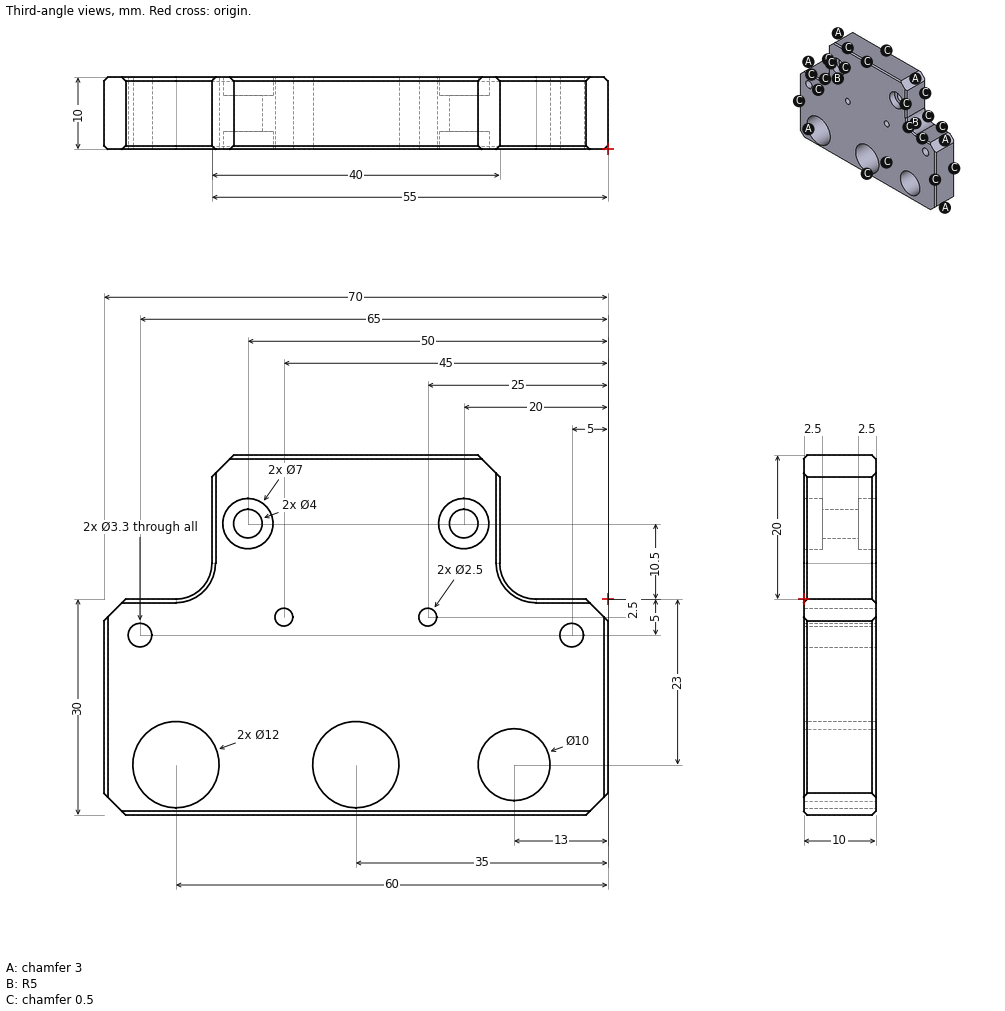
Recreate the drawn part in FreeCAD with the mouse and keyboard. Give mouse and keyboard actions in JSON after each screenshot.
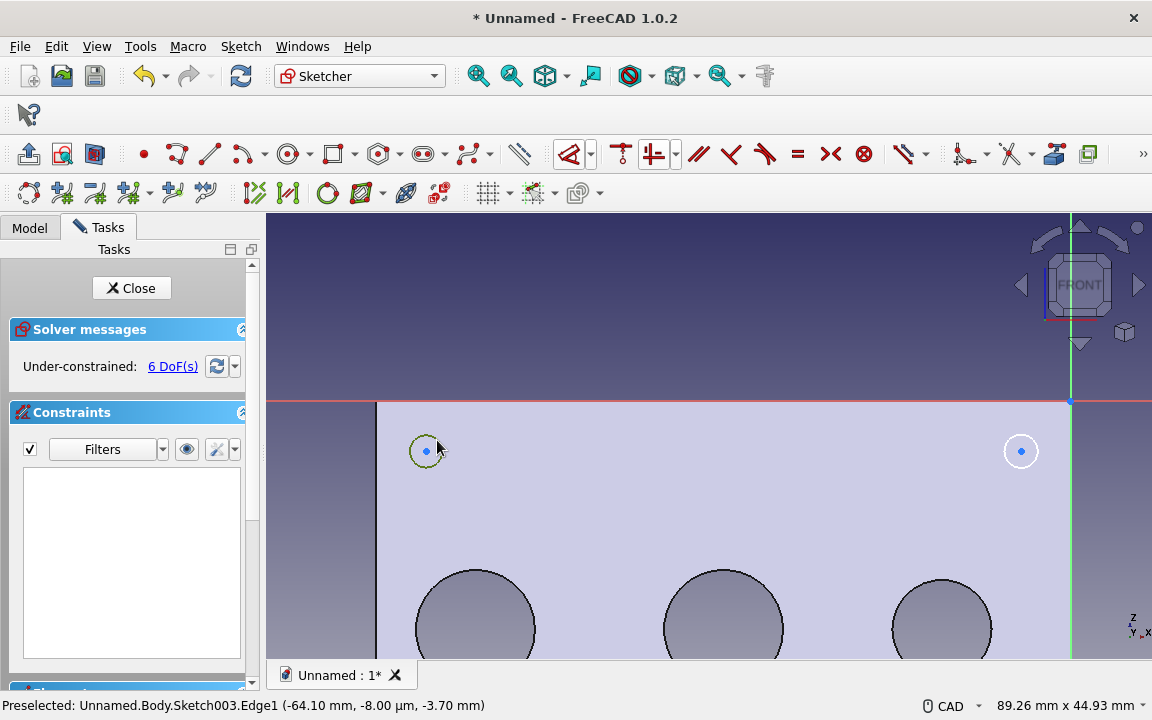
{"action": "scroll", "coordinate": [438, 440], "scroll_direction": "down", "scroll_amount": 2}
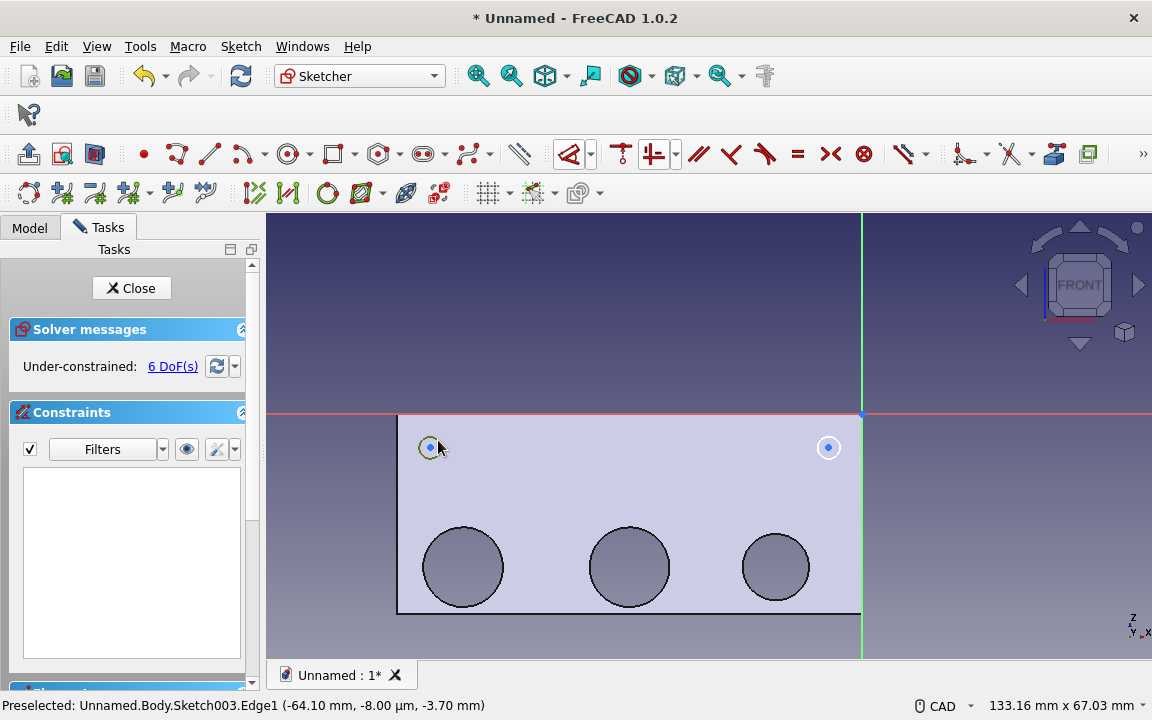
{"action": "scroll", "coordinate": [837, 440], "scroll_direction": "up", "scroll_amount": 2}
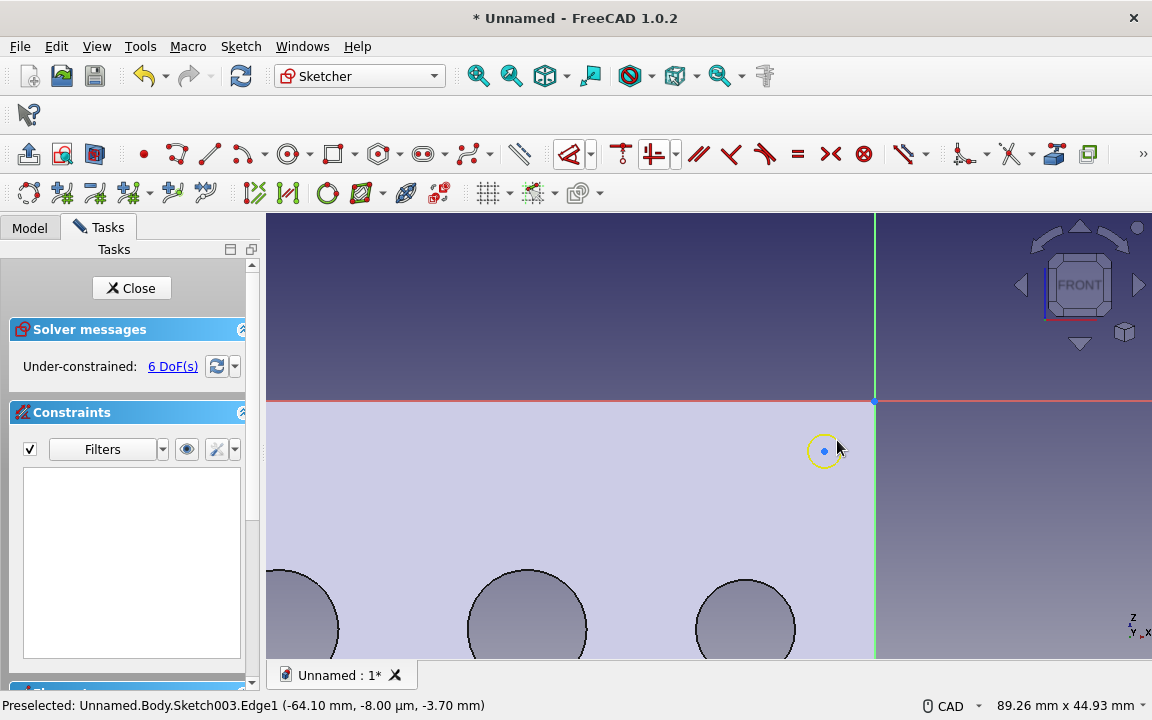
{"action": "left_click", "coordinate": [836, 440]}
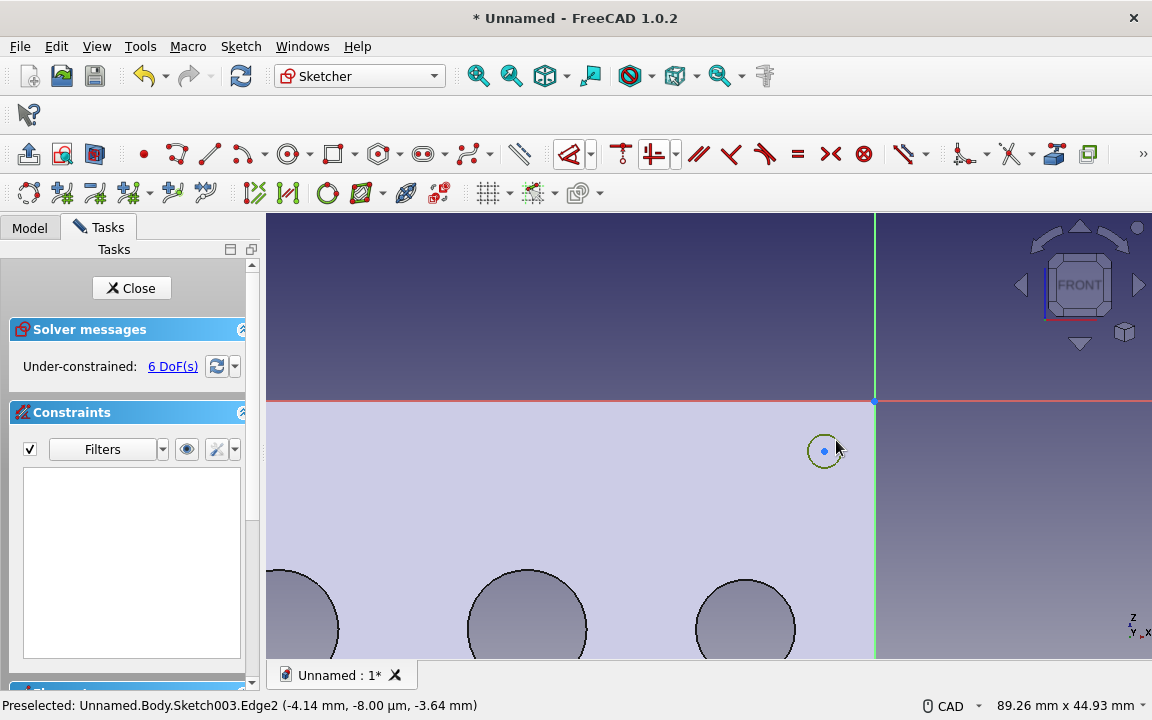
{"action": "left_click", "coordinate": [798, 154]}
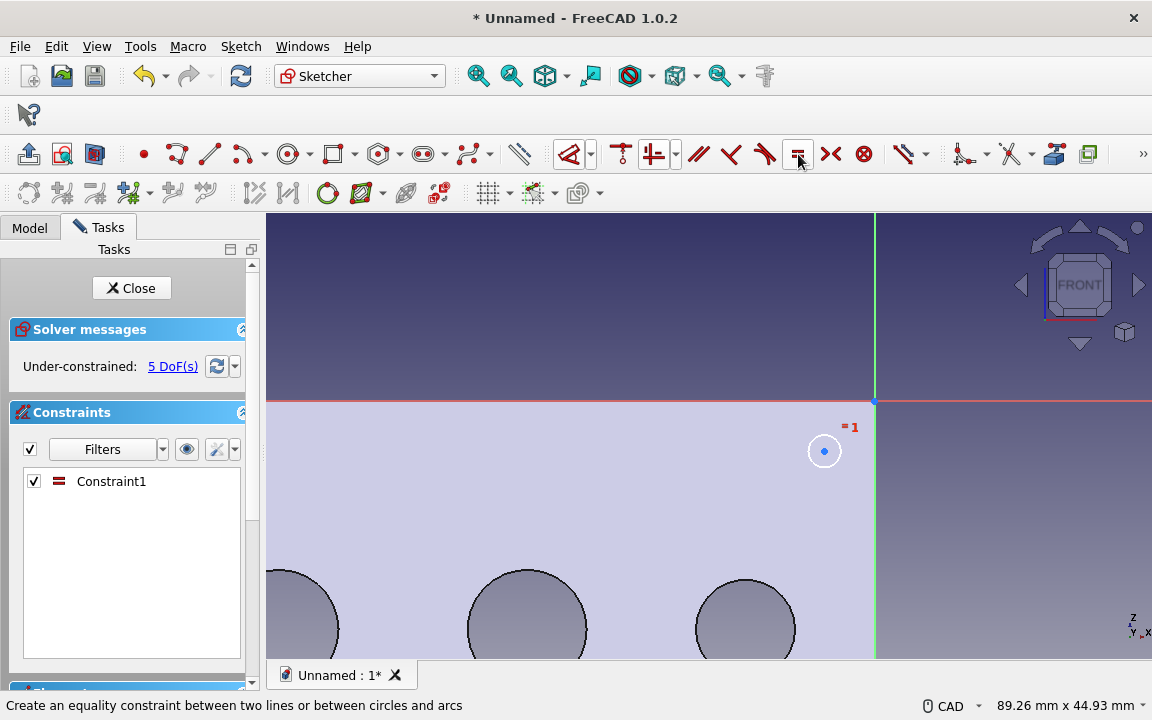
{"action": "scroll", "coordinate": [837, 440], "scroll_direction": "down", "scroll_amount": 2}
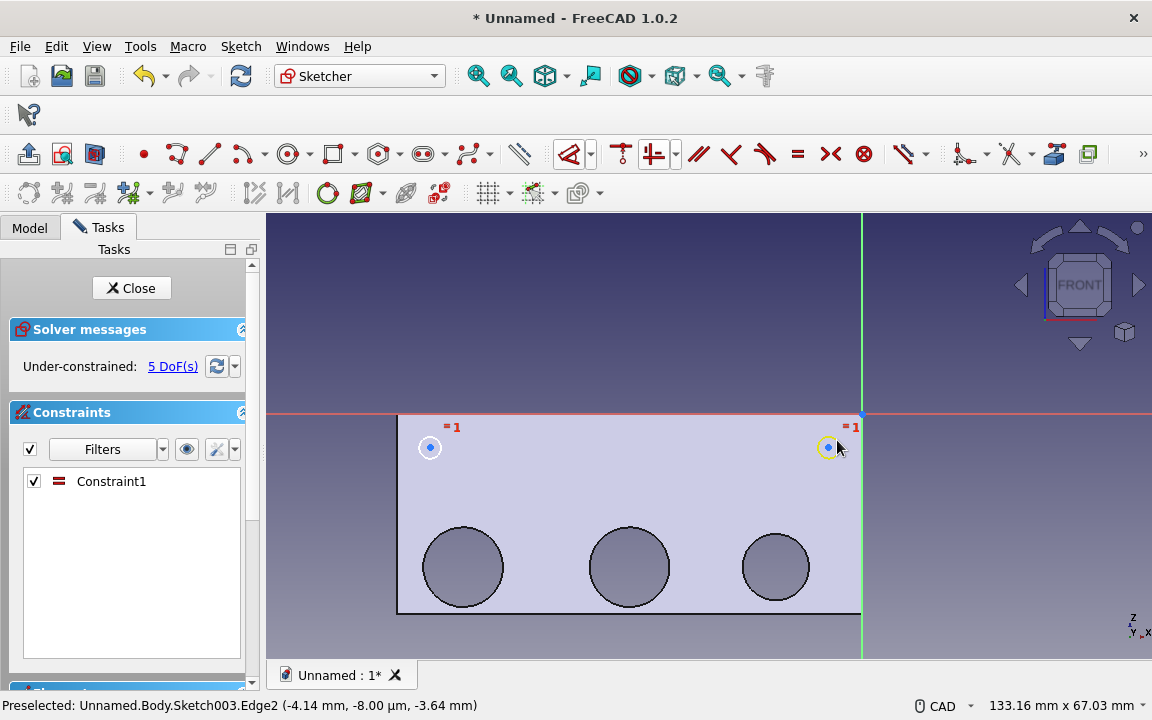
{"action": "left_click", "coordinate": [430, 448]}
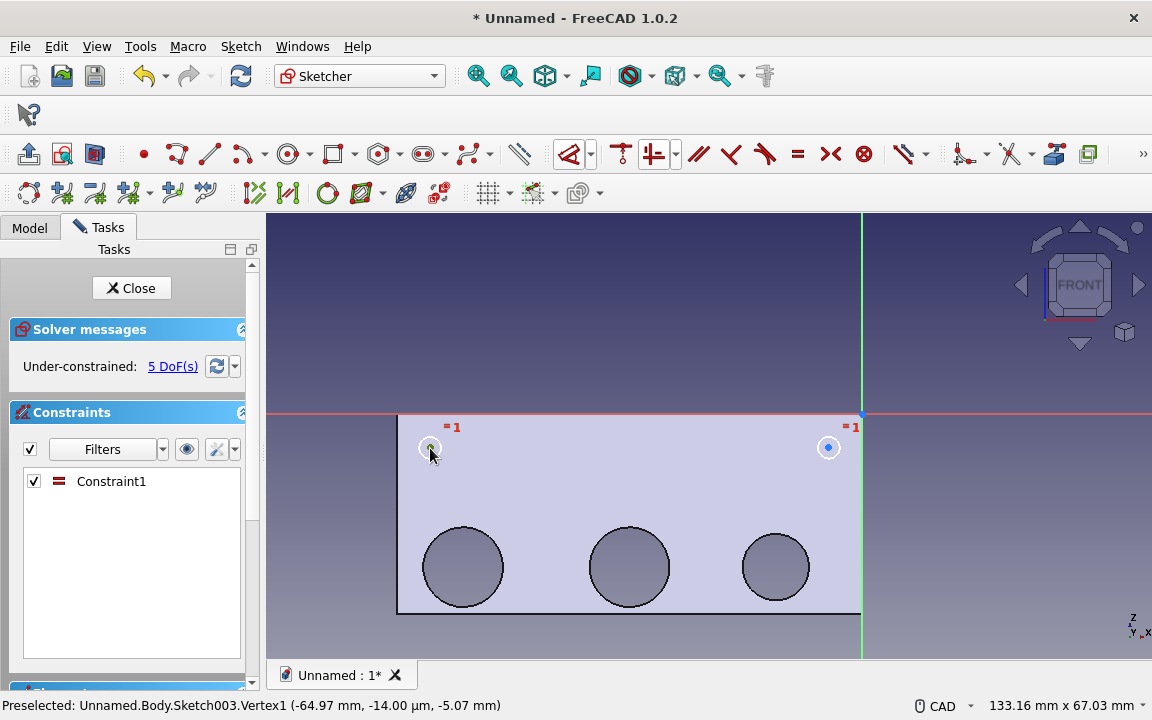
{"action": "left_click", "coordinate": [829, 448]}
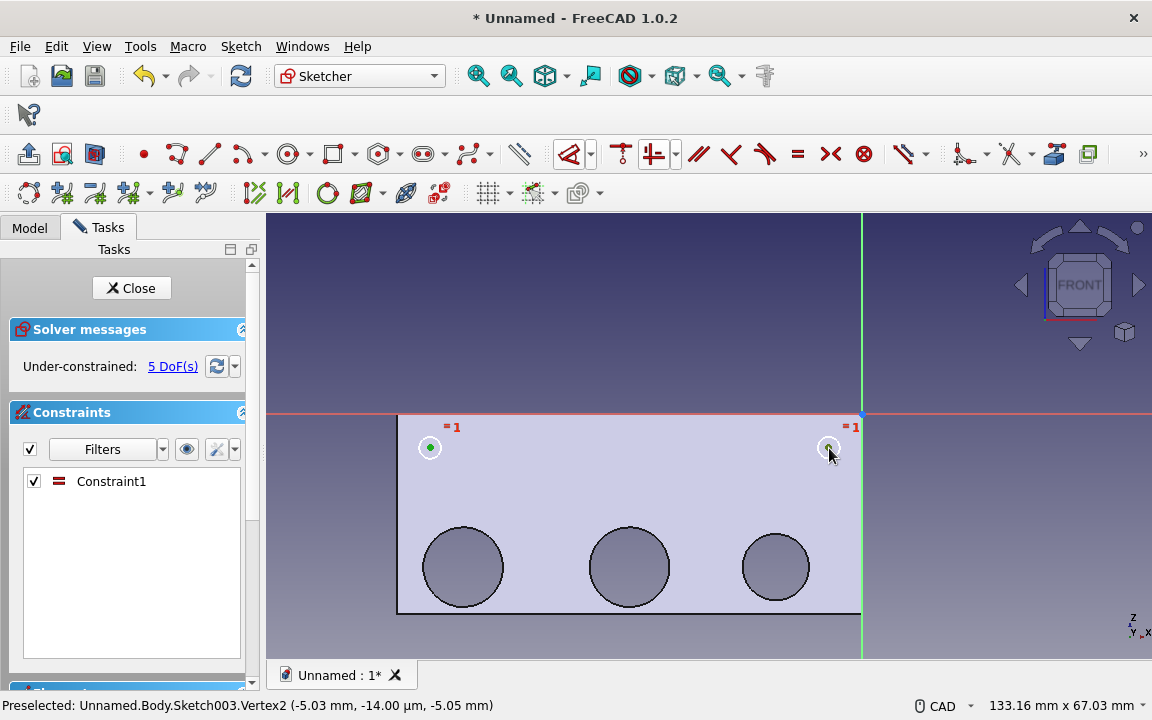
{"action": "left_click", "coordinate": [676, 154]}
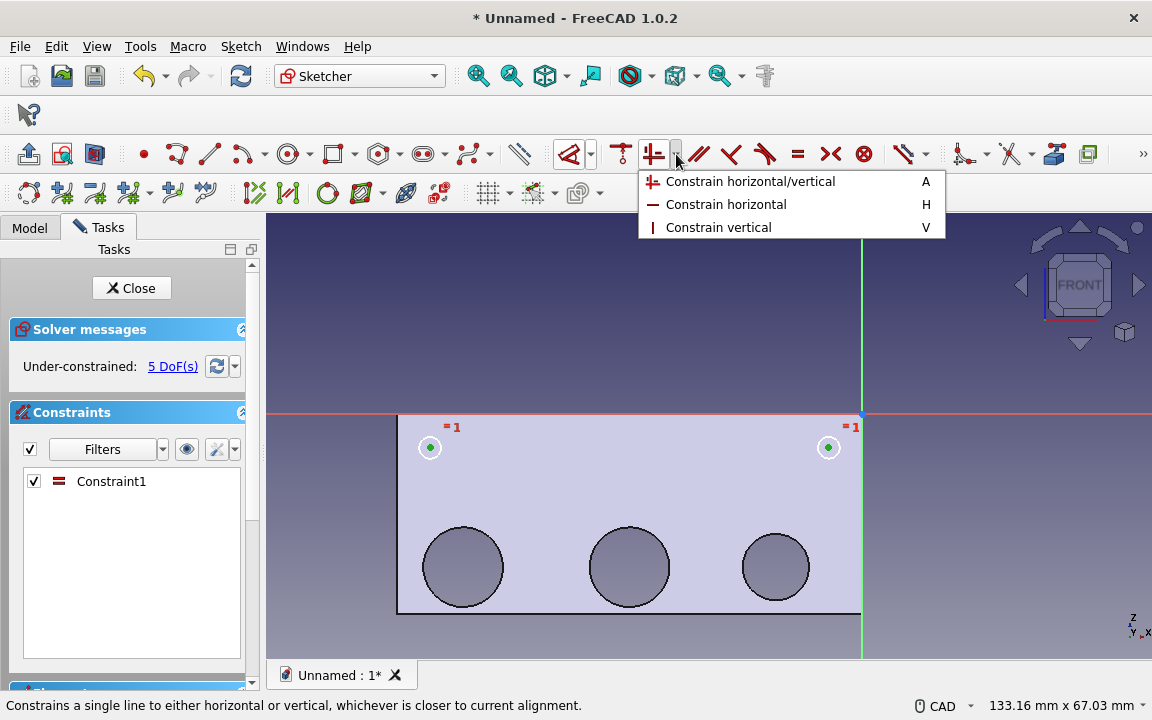
{"action": "left_click", "coordinate": [792, 204]}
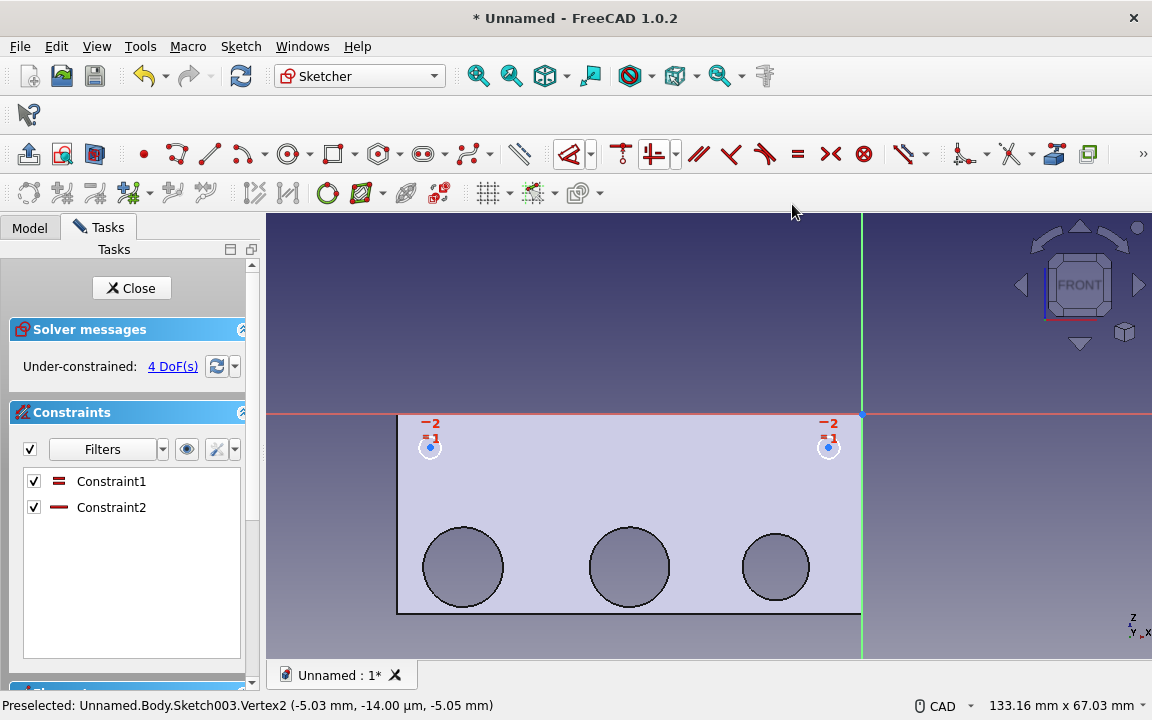
{"action": "scroll", "coordinate": [438, 440], "scroll_direction": "up", "scroll_amount": 3}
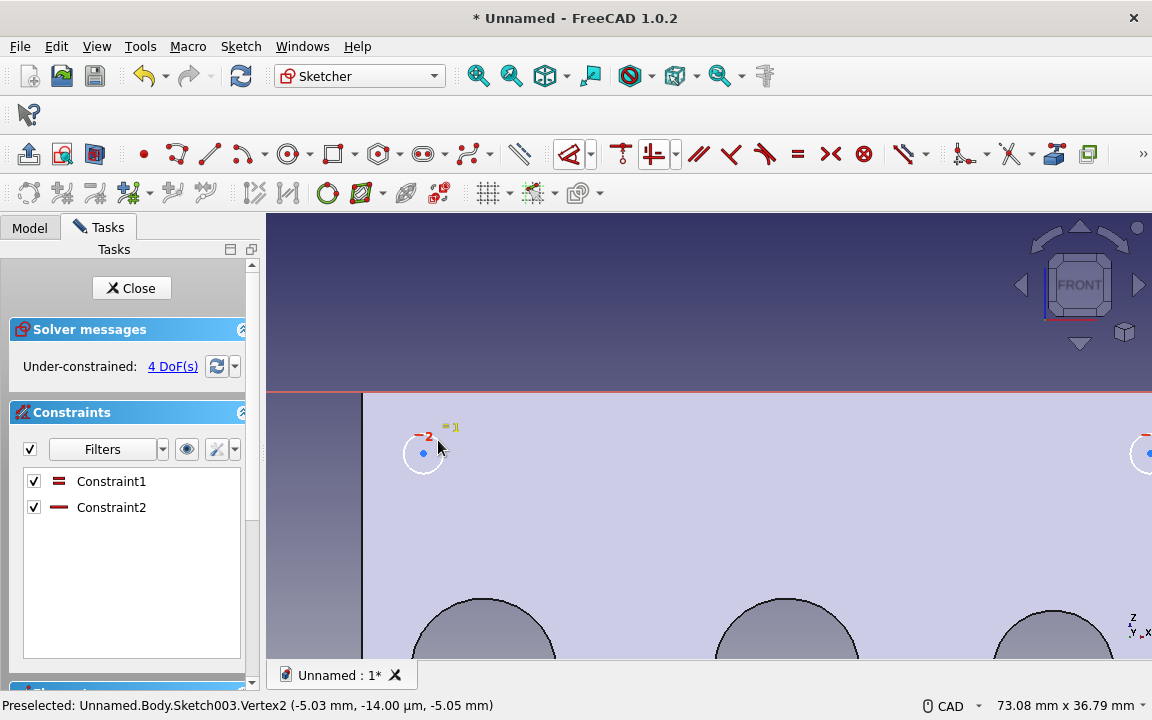
{"action": "left_click", "coordinate": [437, 440]}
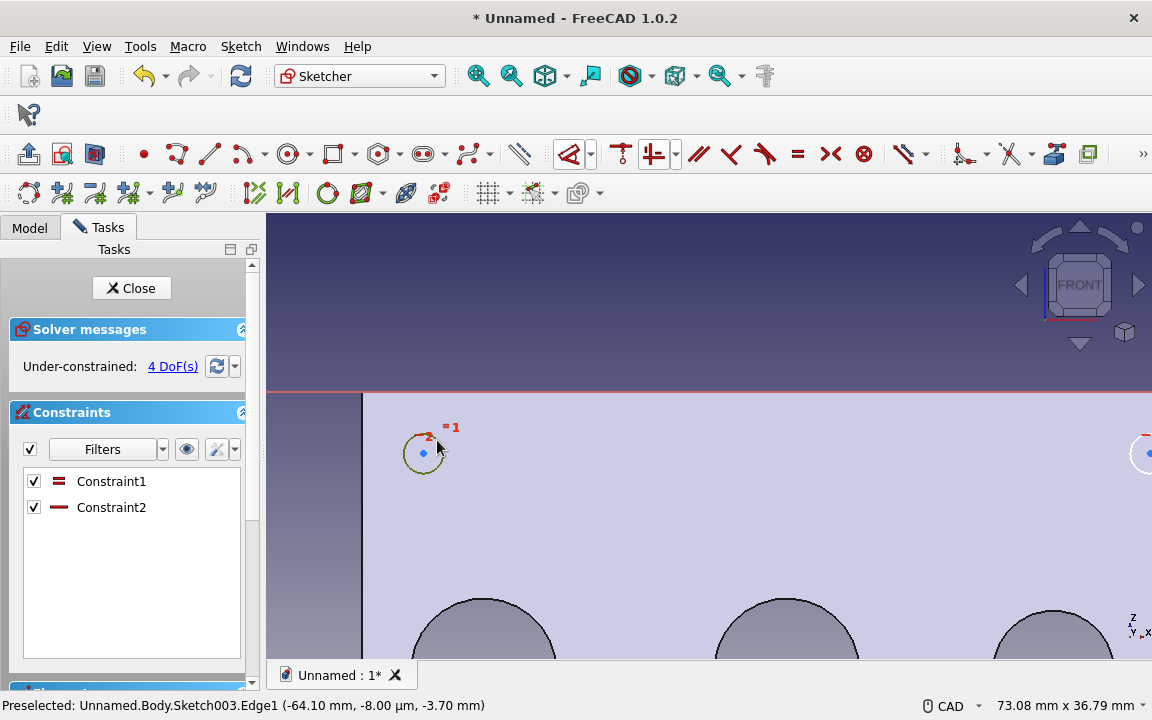
{"action": "left_click", "coordinate": [590, 154]}